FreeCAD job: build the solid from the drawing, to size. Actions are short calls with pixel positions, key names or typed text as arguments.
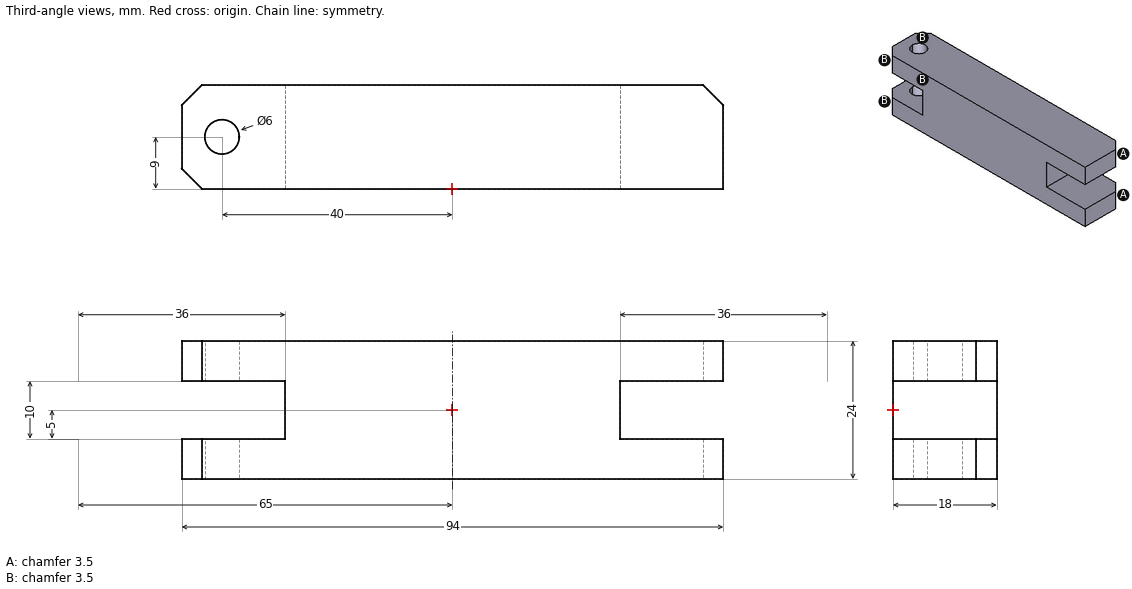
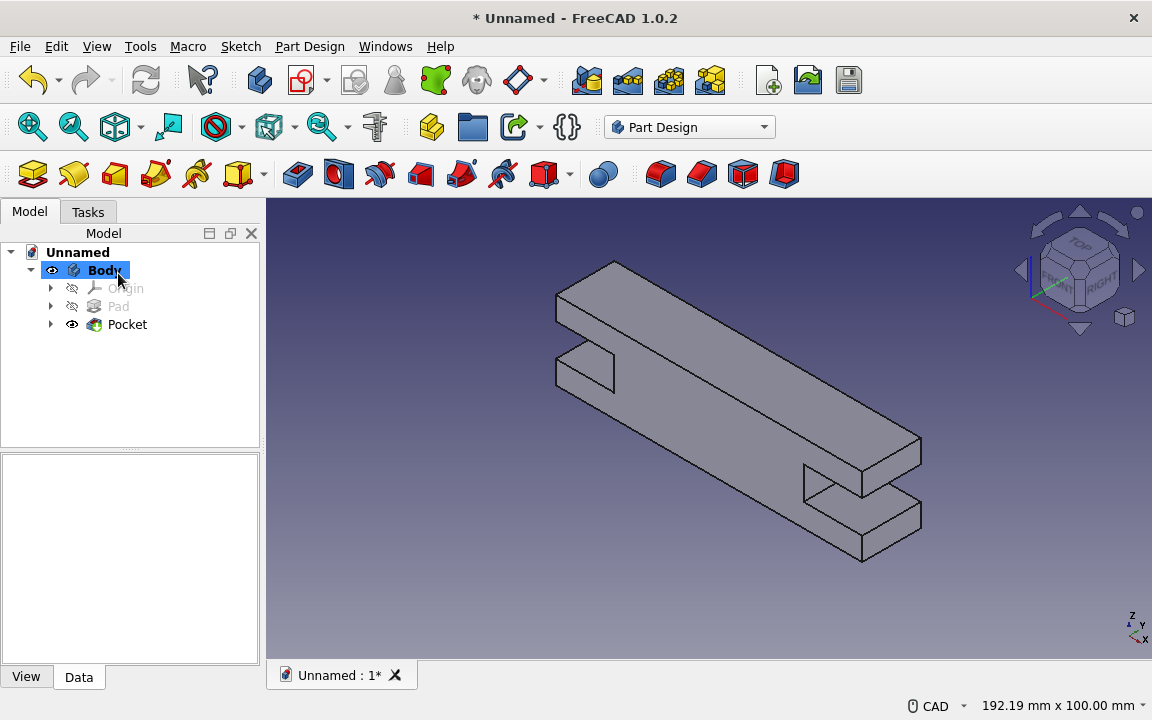
key(2)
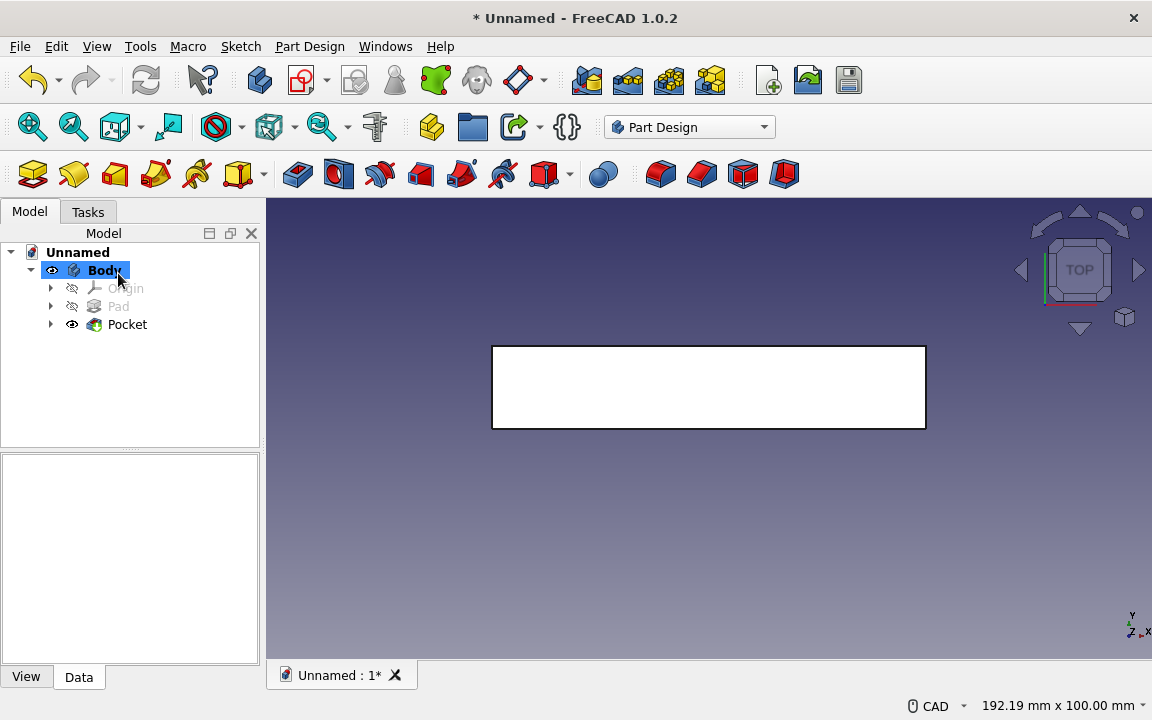
key(1)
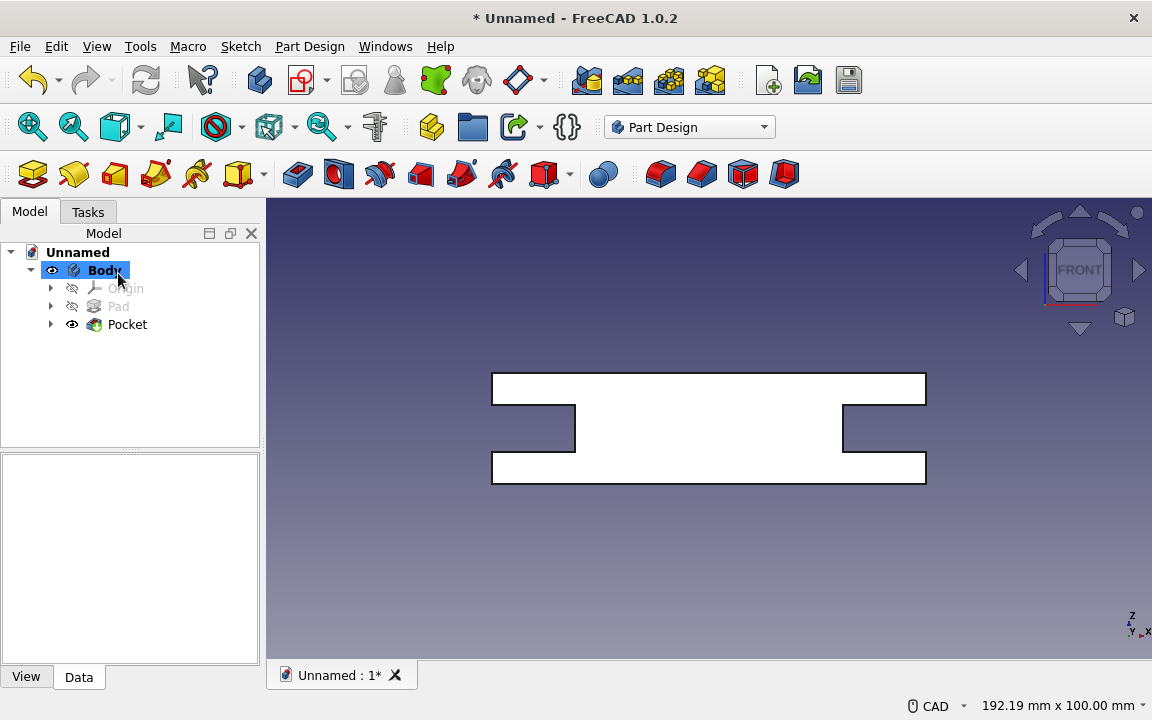
key(3)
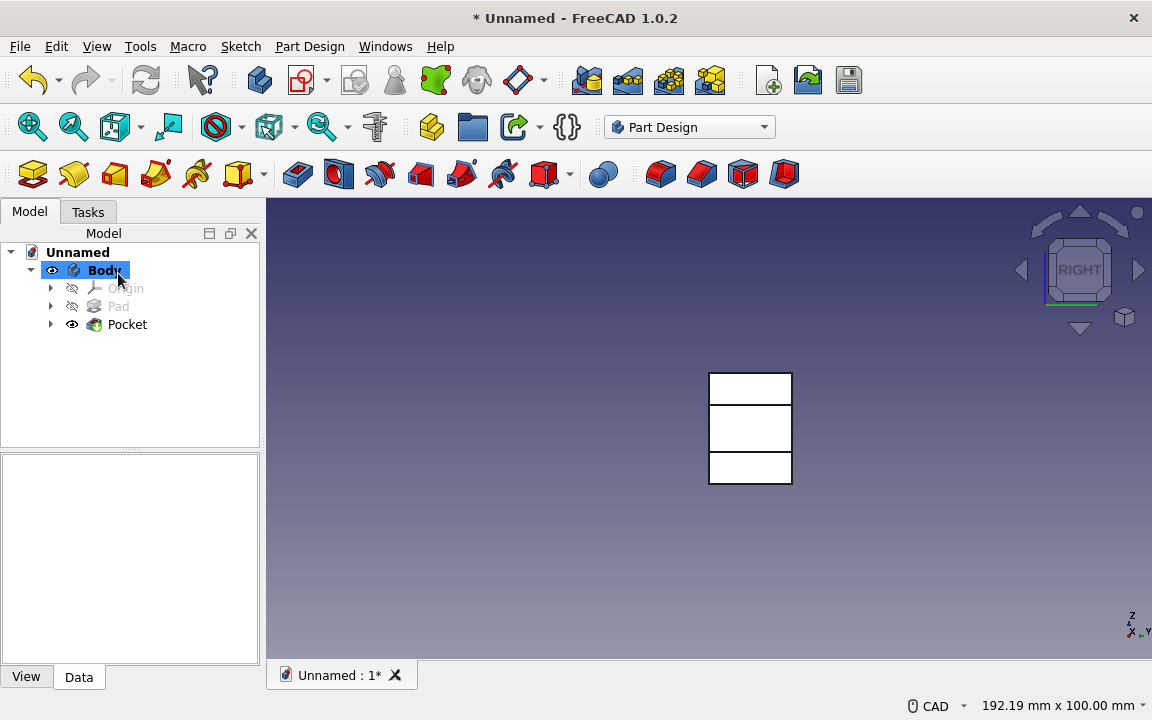
key(v)
key(f)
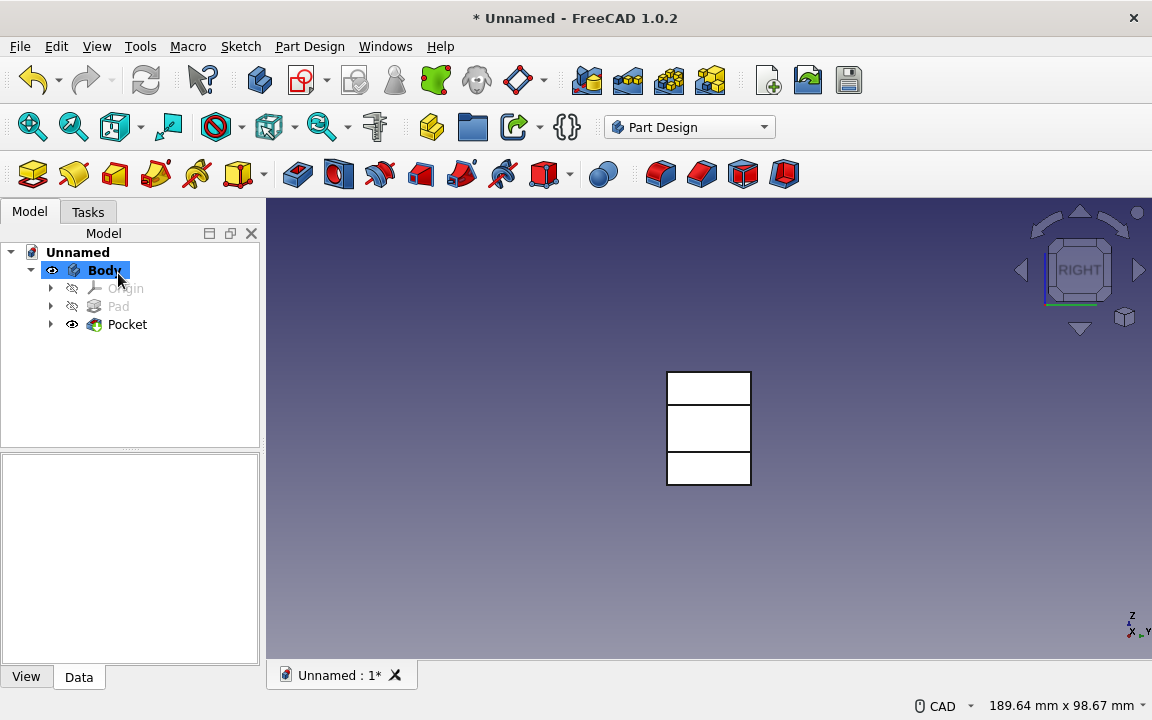
click(751, 467)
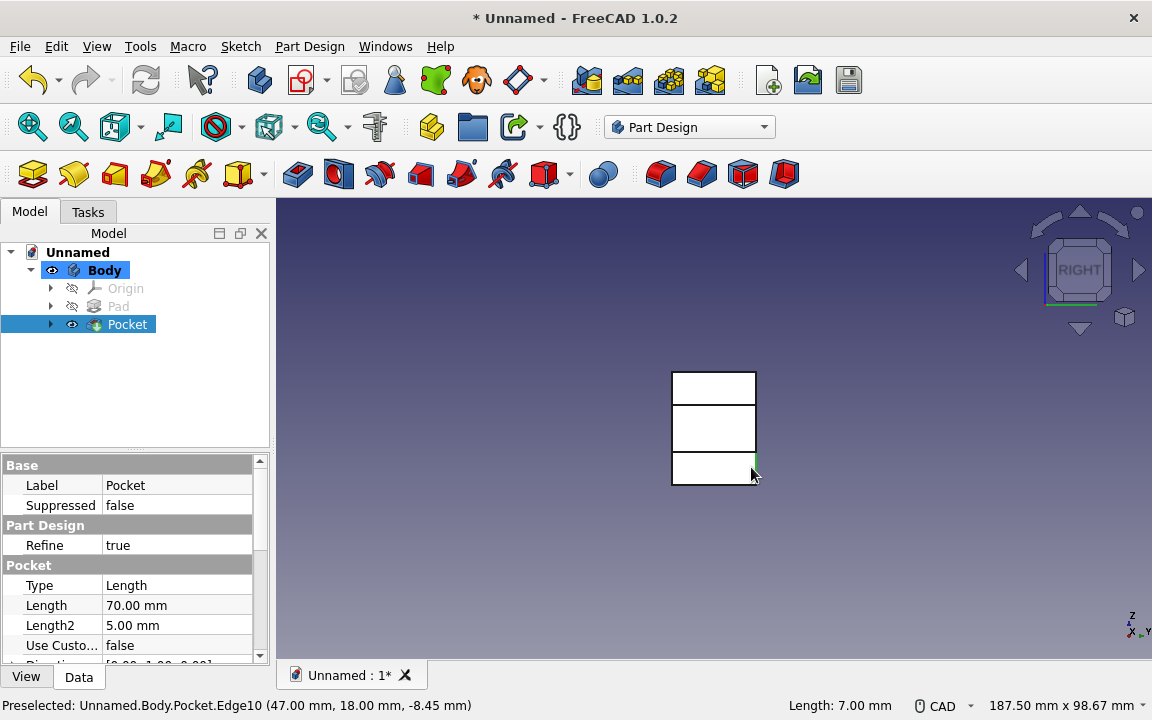
click(756, 388, ctrl)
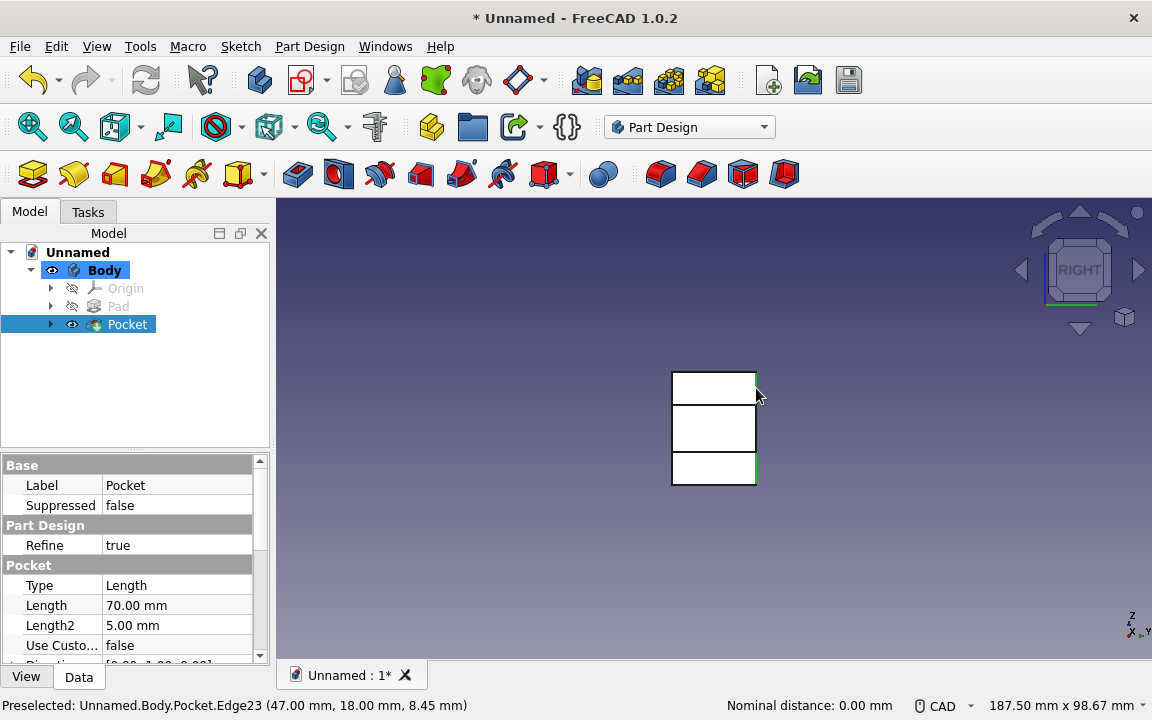
click(702, 174)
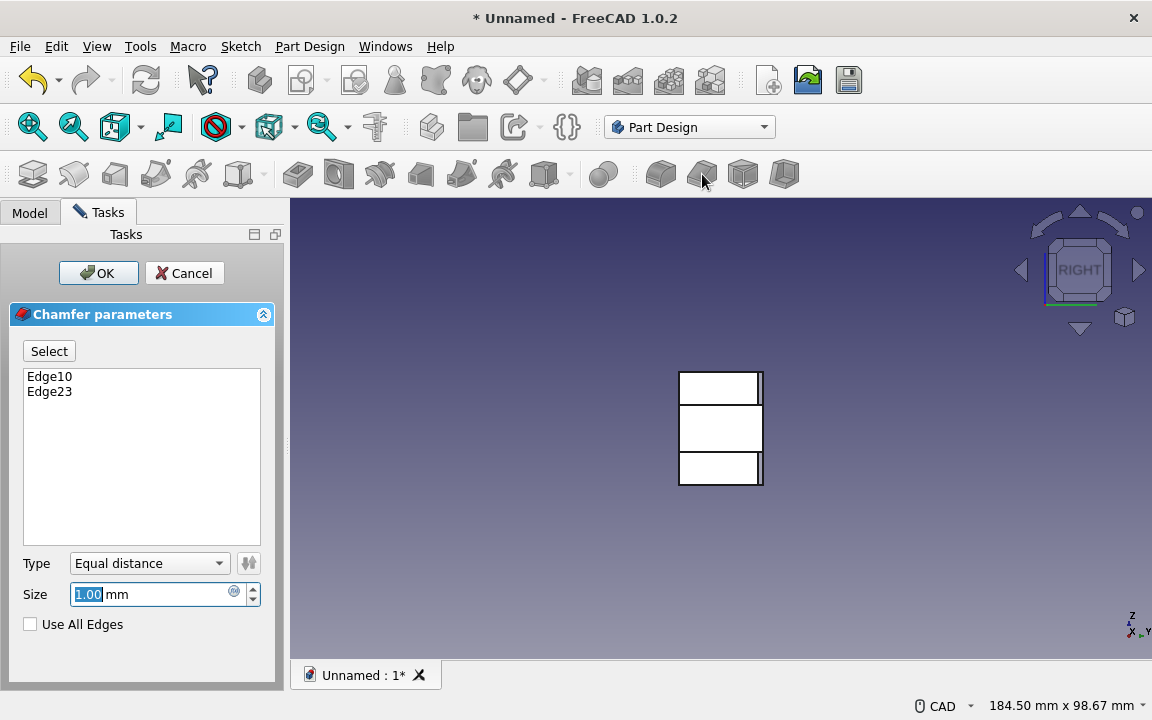
text(3.5)
key(Tab)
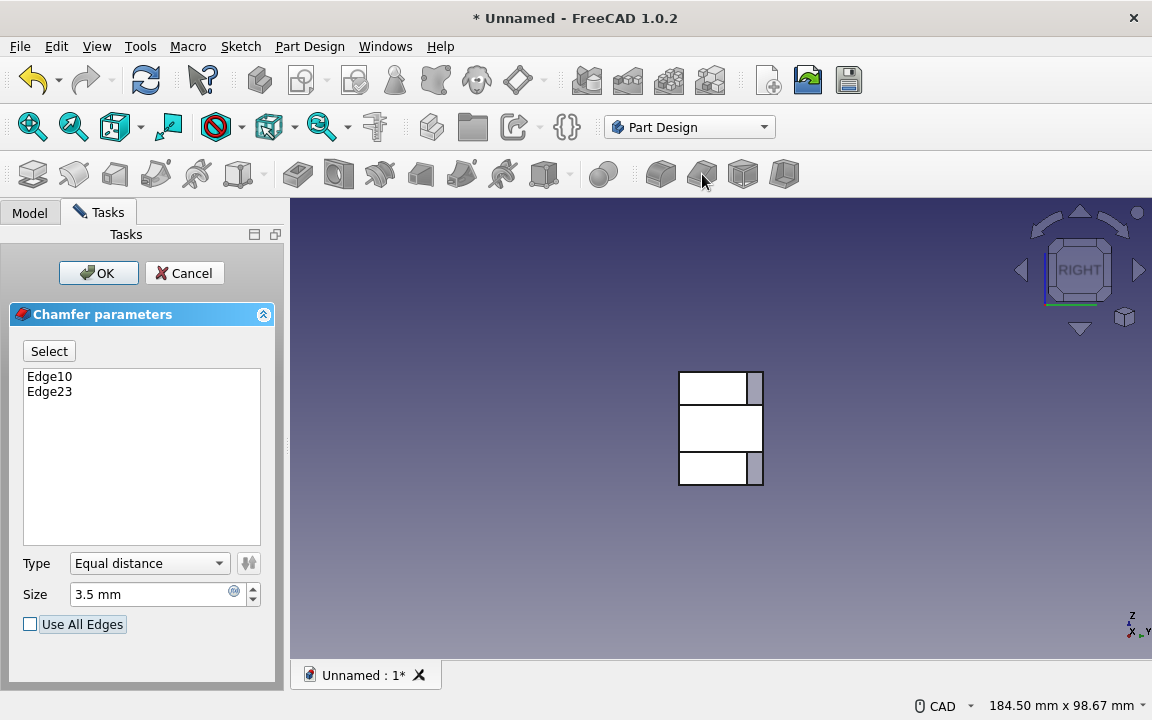
click(99, 273)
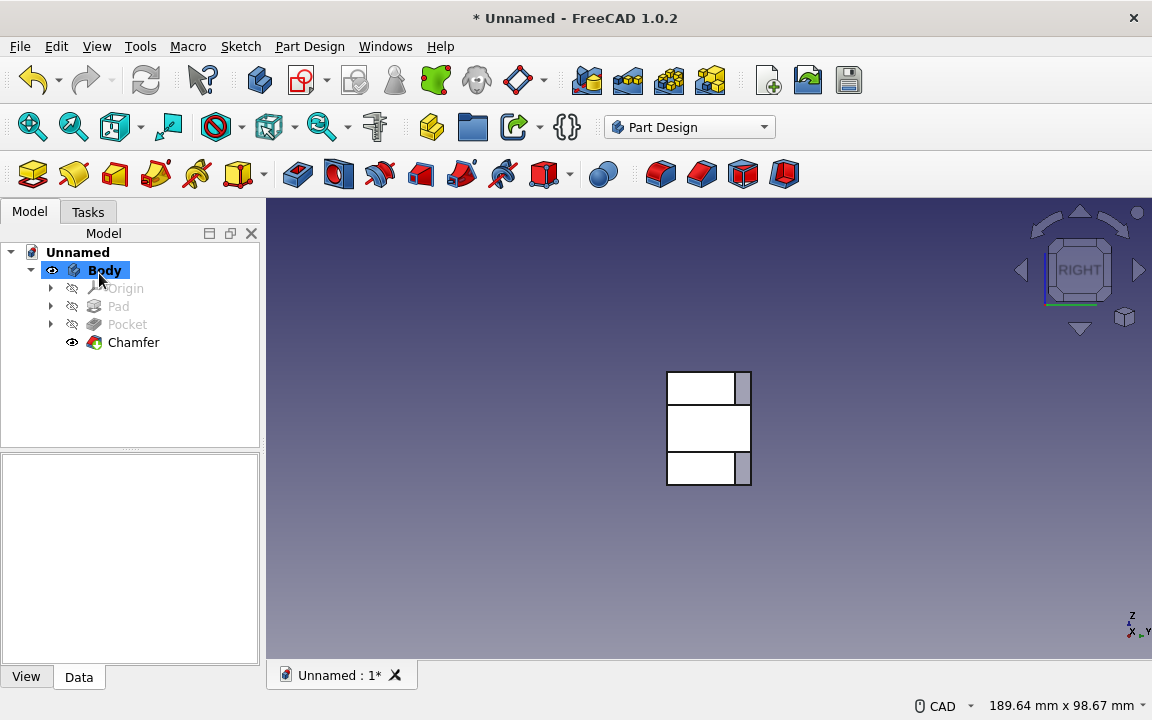
click(33, 128)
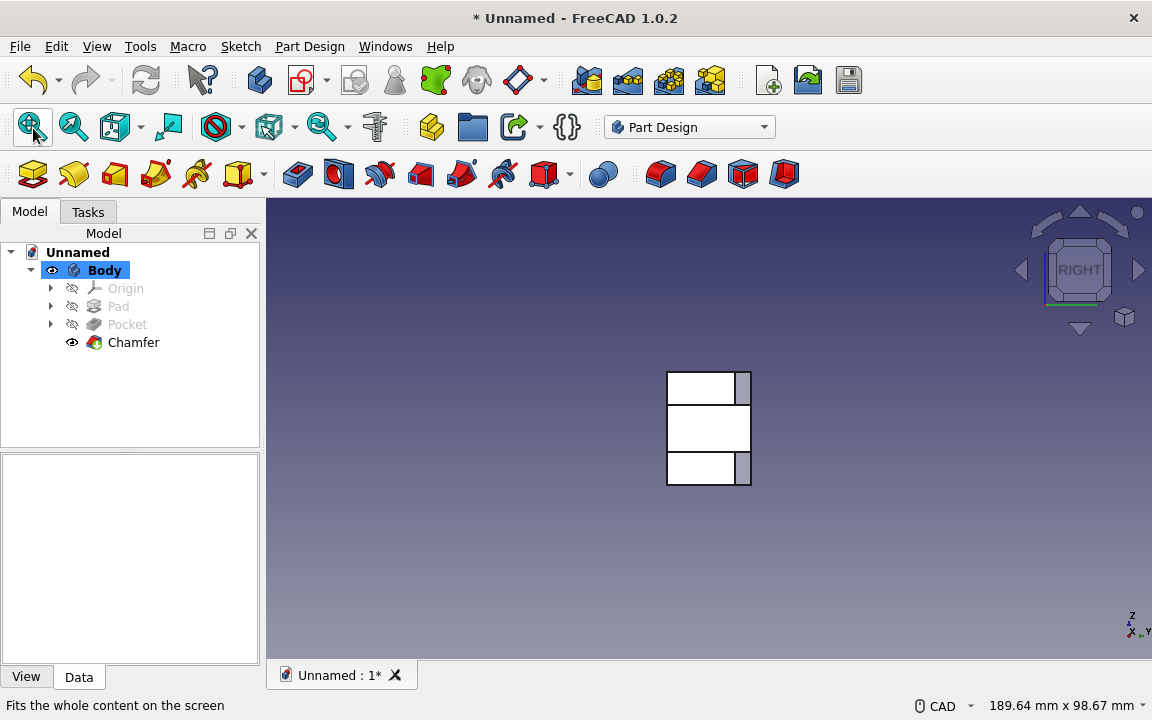
key(0)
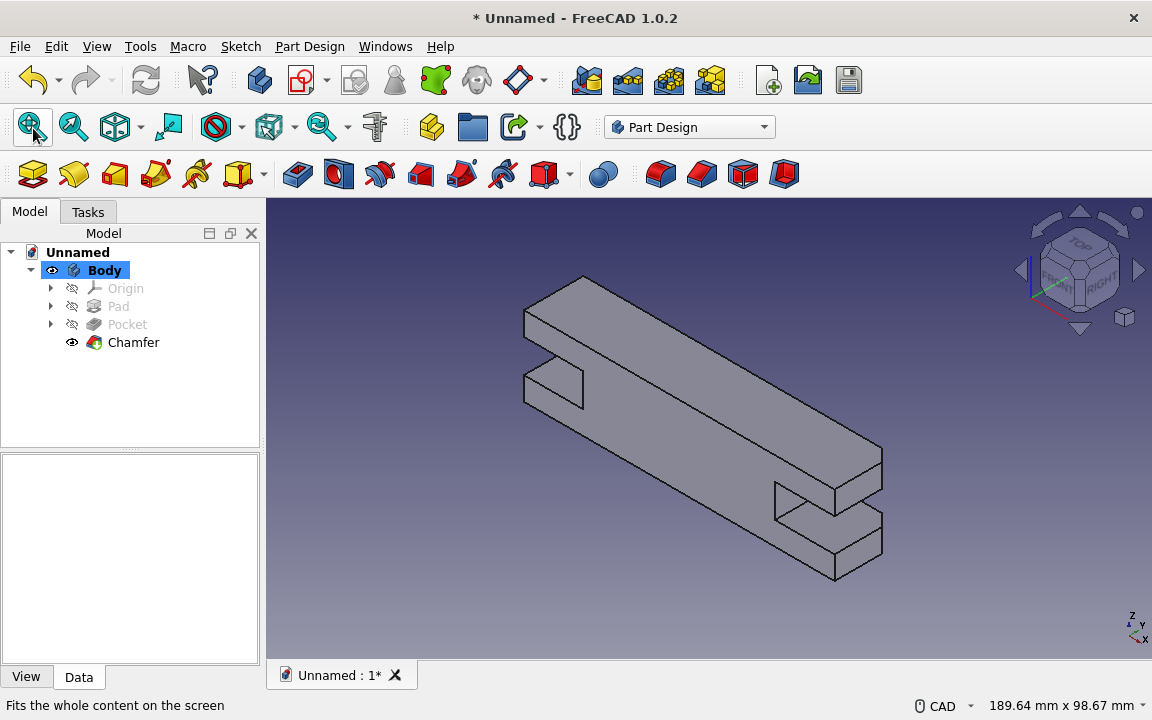
key(2)